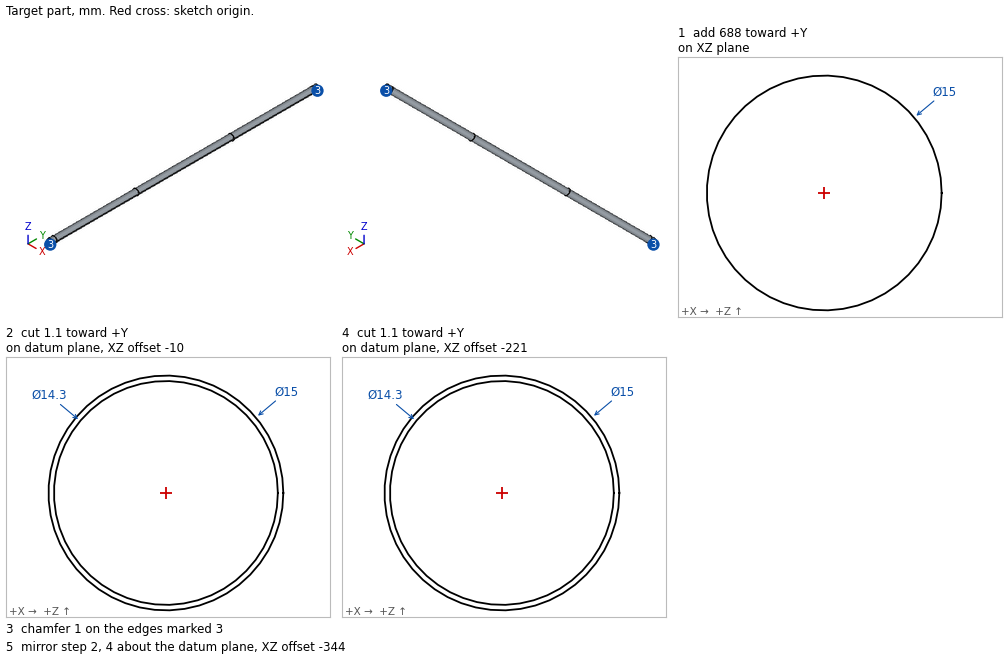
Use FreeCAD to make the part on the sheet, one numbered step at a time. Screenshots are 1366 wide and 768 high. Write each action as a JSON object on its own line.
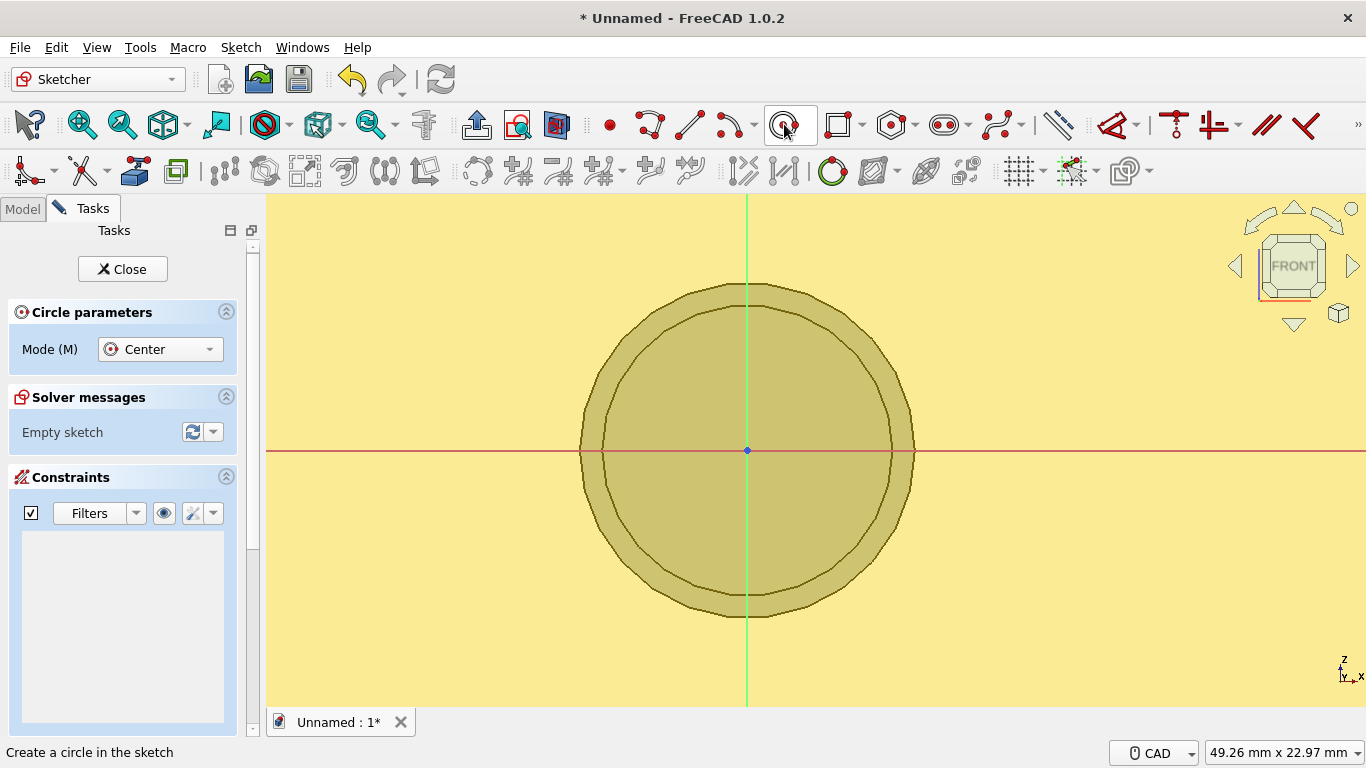
{"action": "left_click", "coordinate": [747, 451]}
{"action": "mouse_move", "coordinate": [866, 332]}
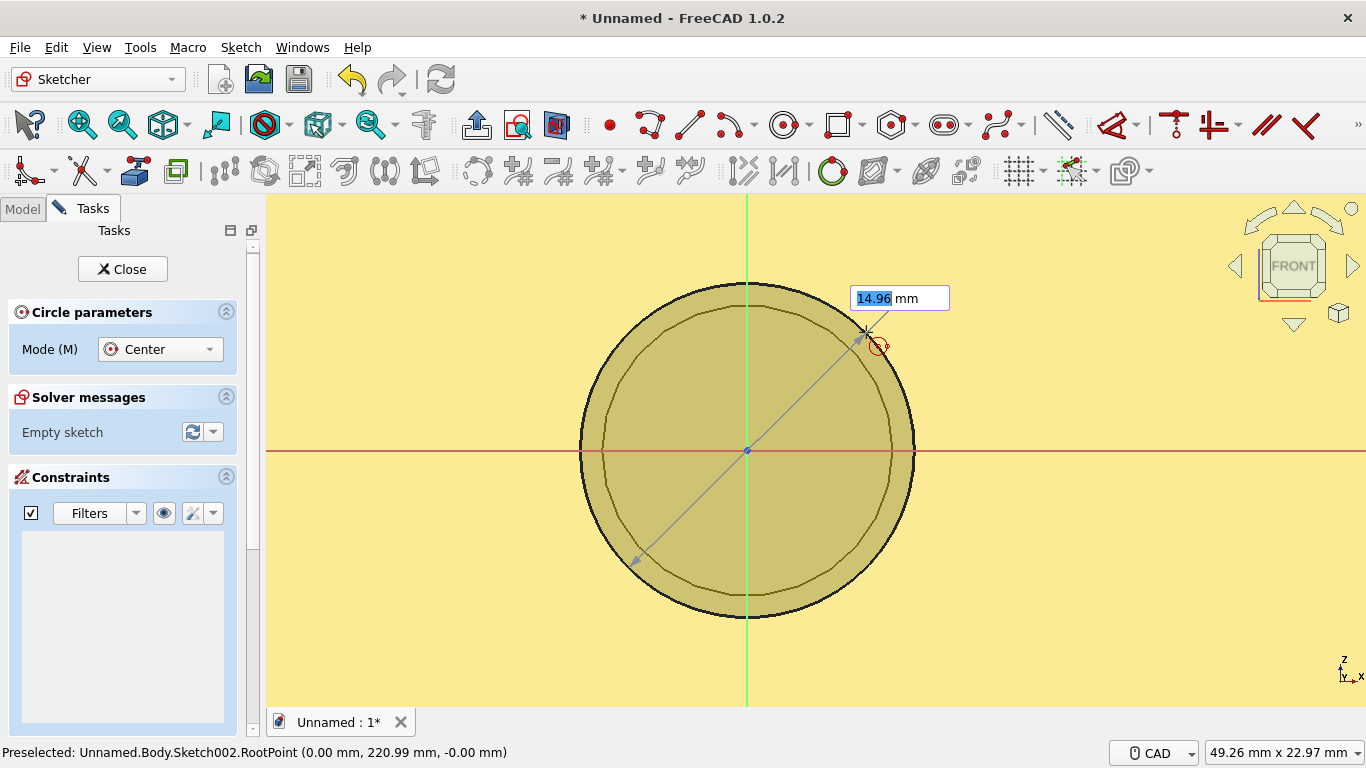
{"action": "type", "text": "15"}
{"action": "key", "text": "Return"}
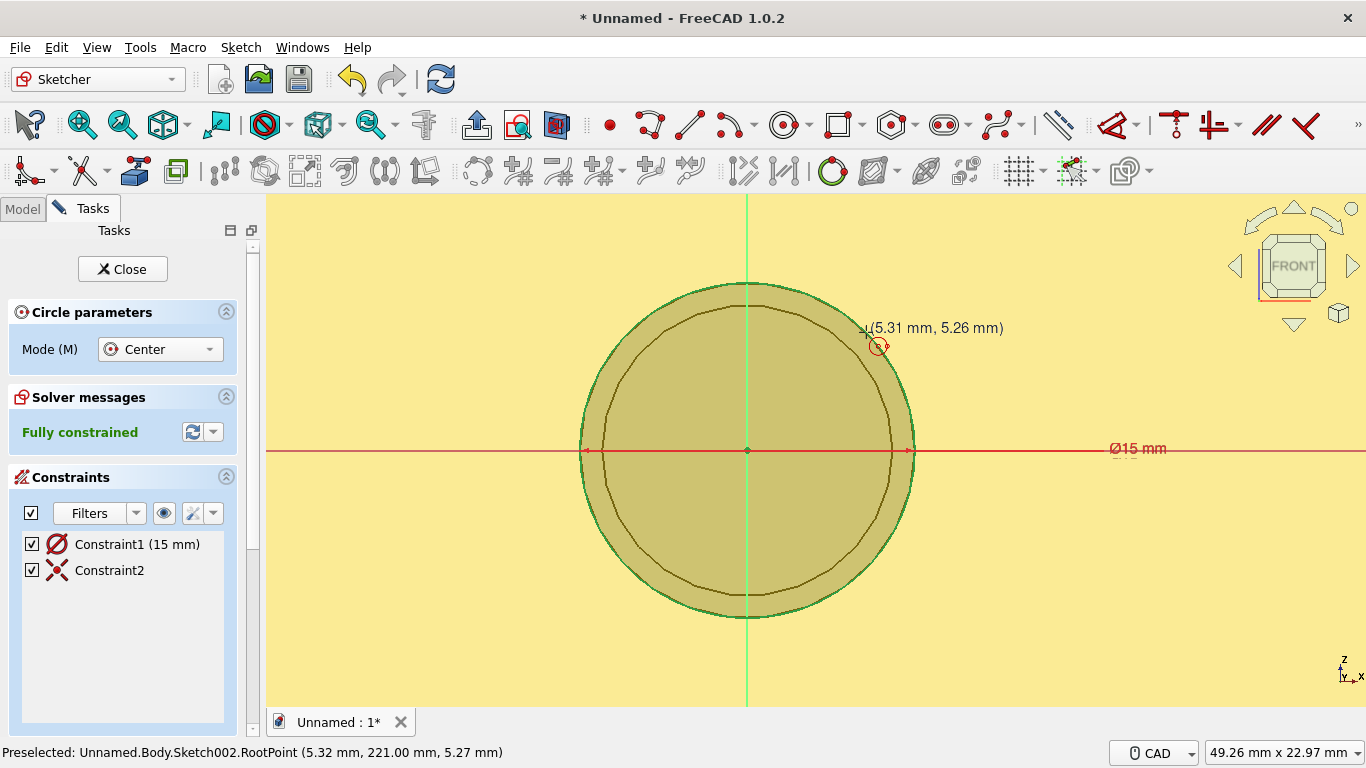
{"action": "left_click", "coordinate": [747, 451]}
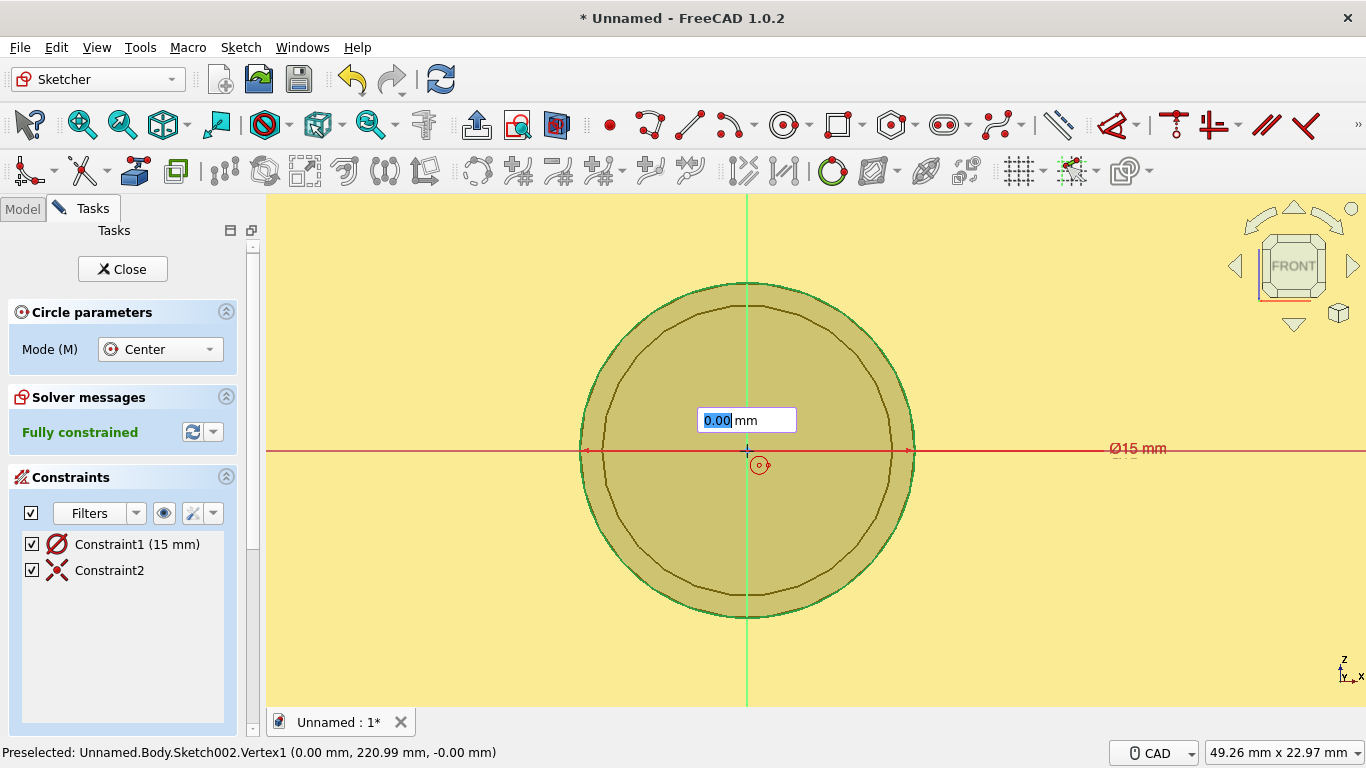
{"action": "scroll", "coordinate": [802, 301], "scroll_direction": "up", "scroll_amount": 4}
{"action": "mouse_move", "coordinate": [801, 300]}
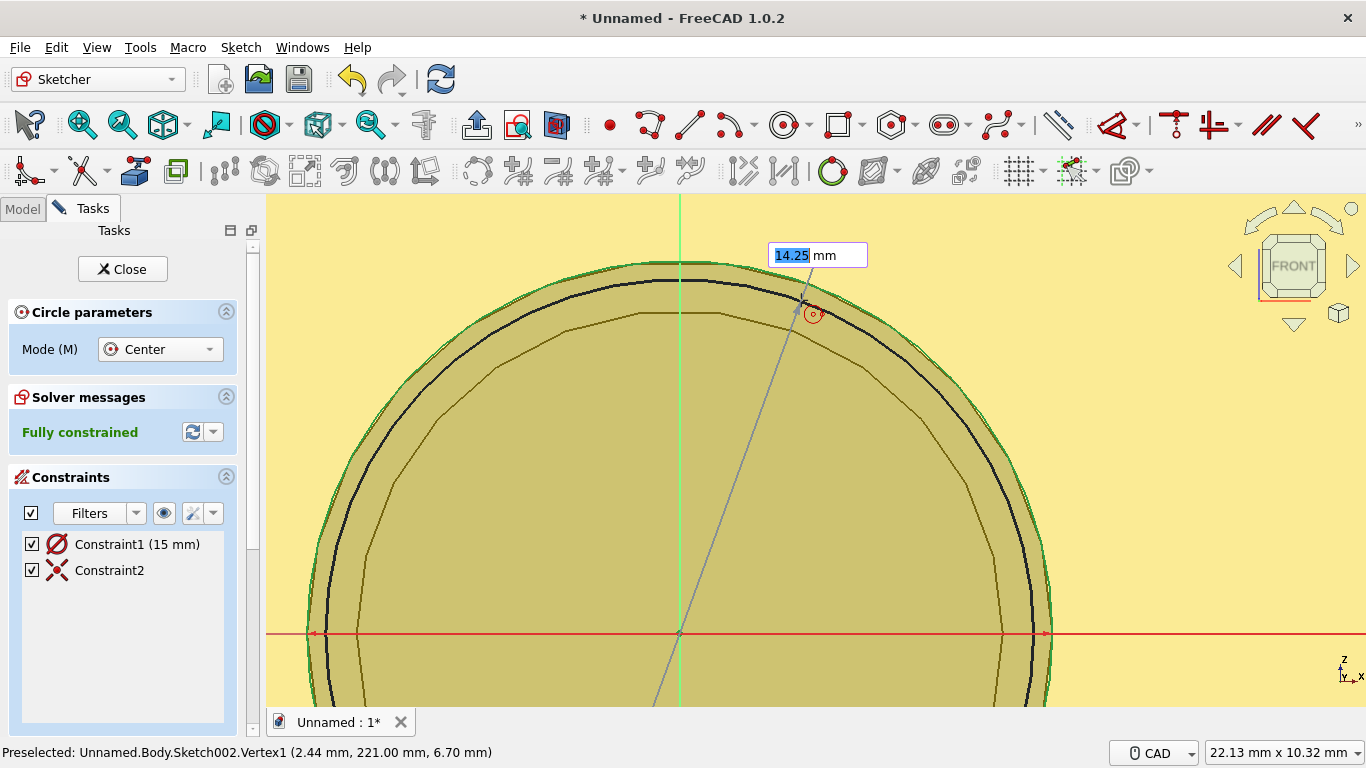
{"action": "type", "text": "14.3"}
{"action": "key", "text": "Return"}
{"action": "key", "text": "Escape"}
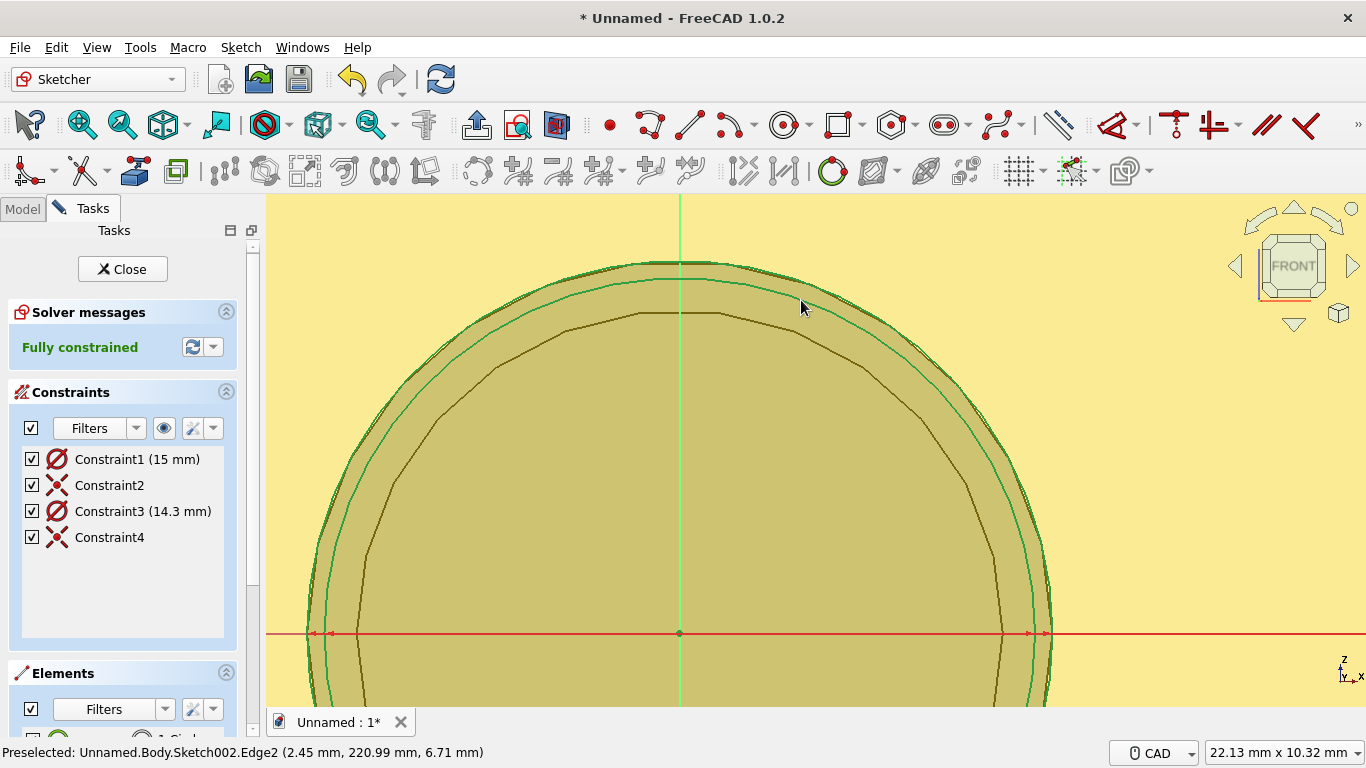
{"action": "left_click", "coordinate": [123, 269]}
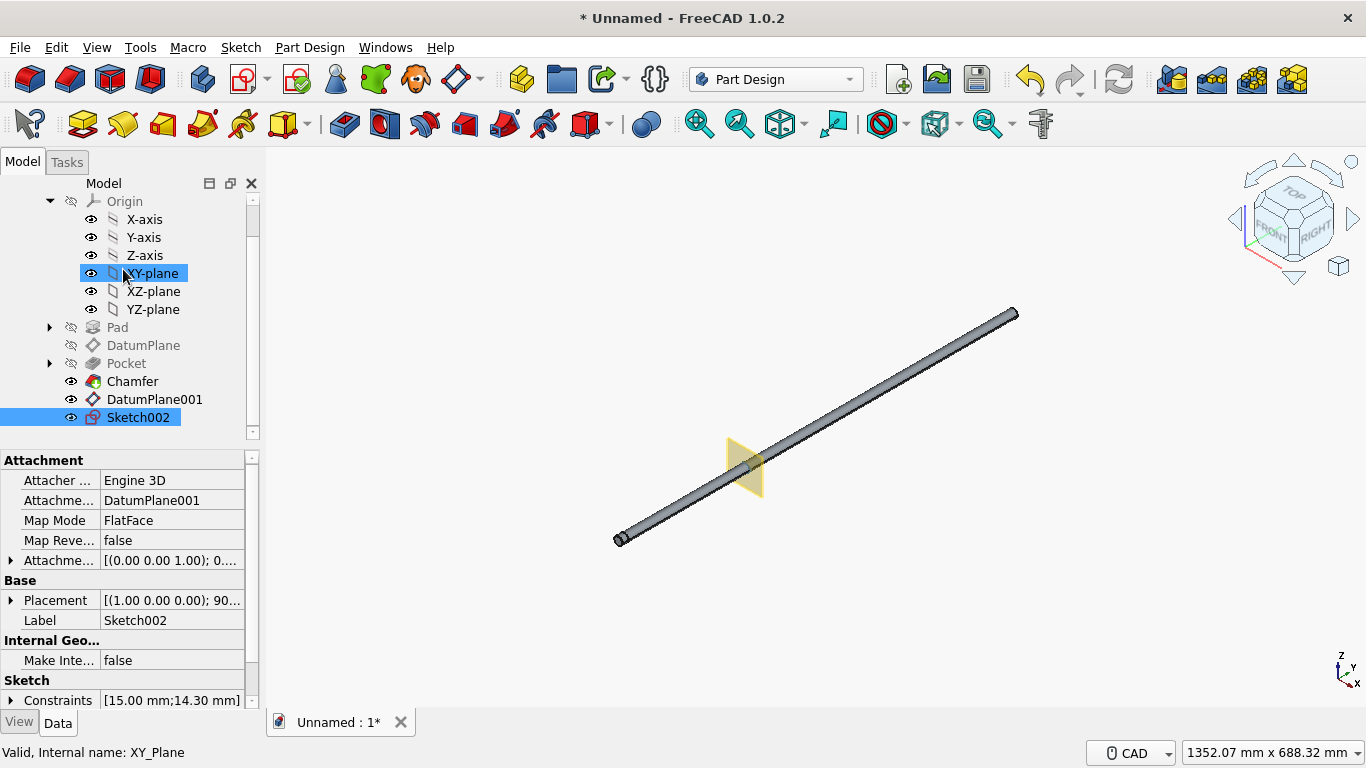
{"action": "left_click", "coordinate": [346, 124]}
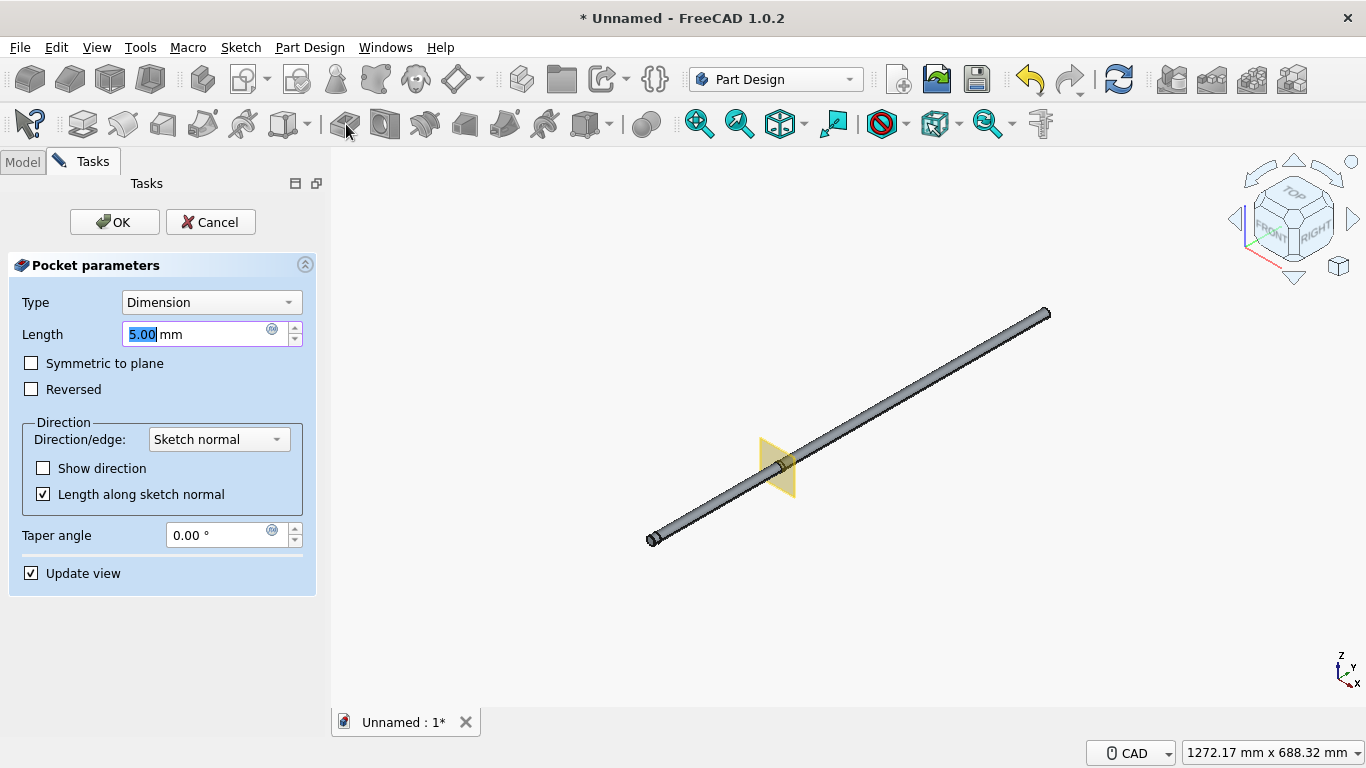
{"action": "type", "text": "1.1"}
{"action": "key", "text": "Tab"}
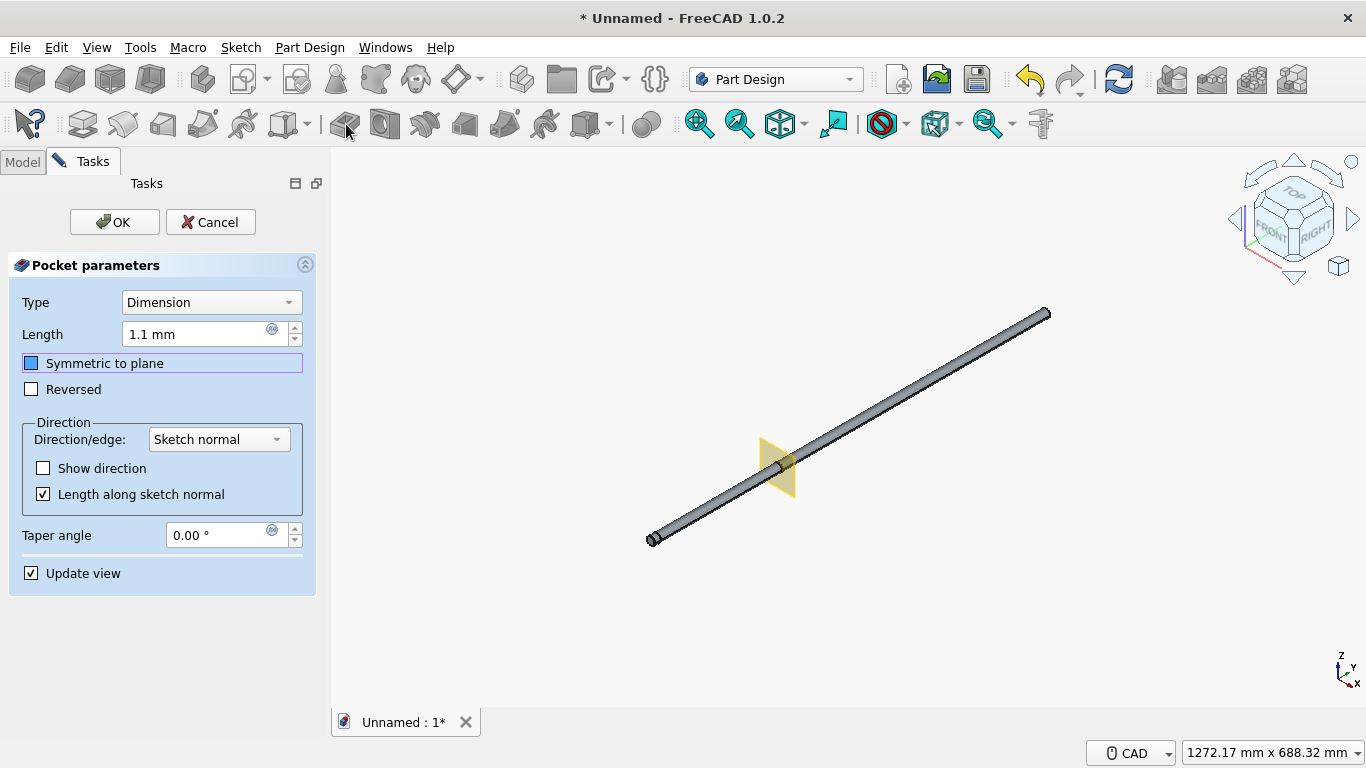
{"action": "left_click", "coordinate": [115, 222]}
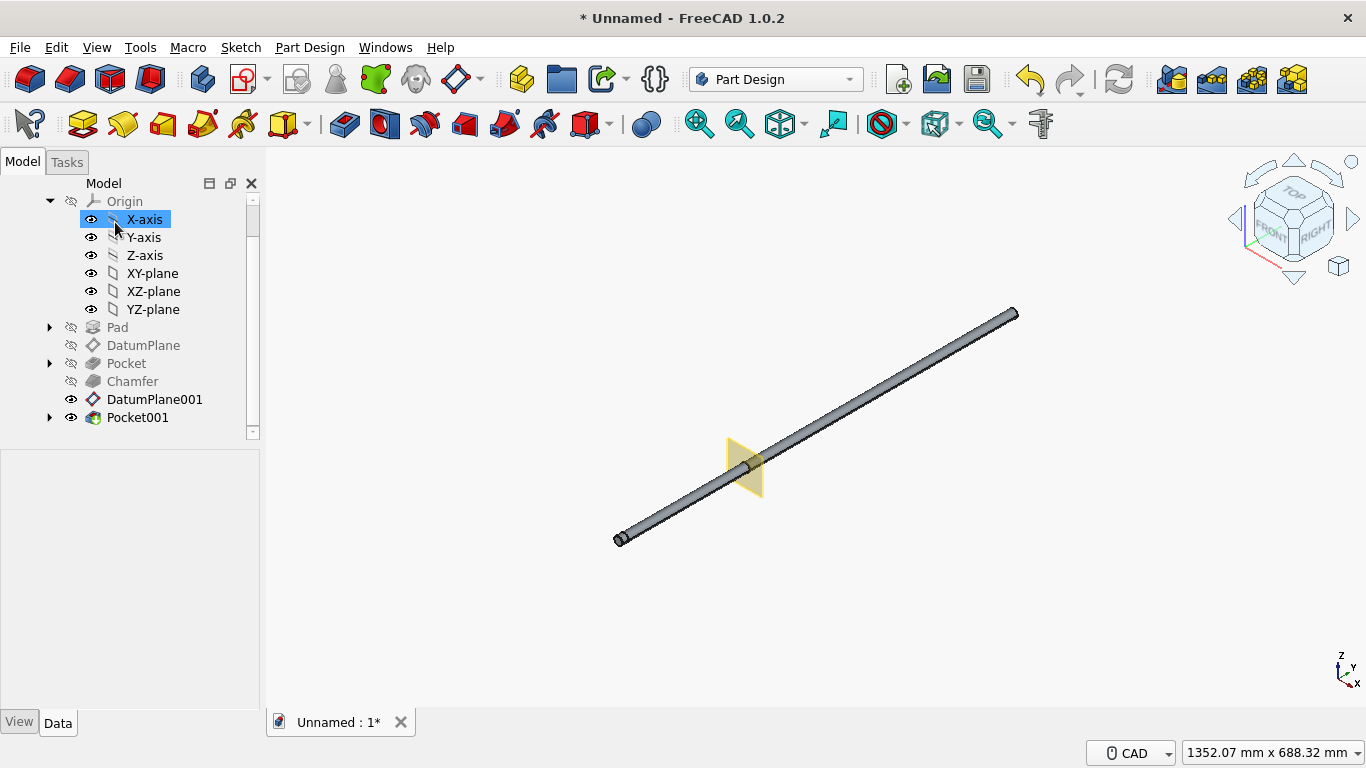
{"action": "left_click", "coordinate": [116, 399]}
{"action": "key", "text": "space"}